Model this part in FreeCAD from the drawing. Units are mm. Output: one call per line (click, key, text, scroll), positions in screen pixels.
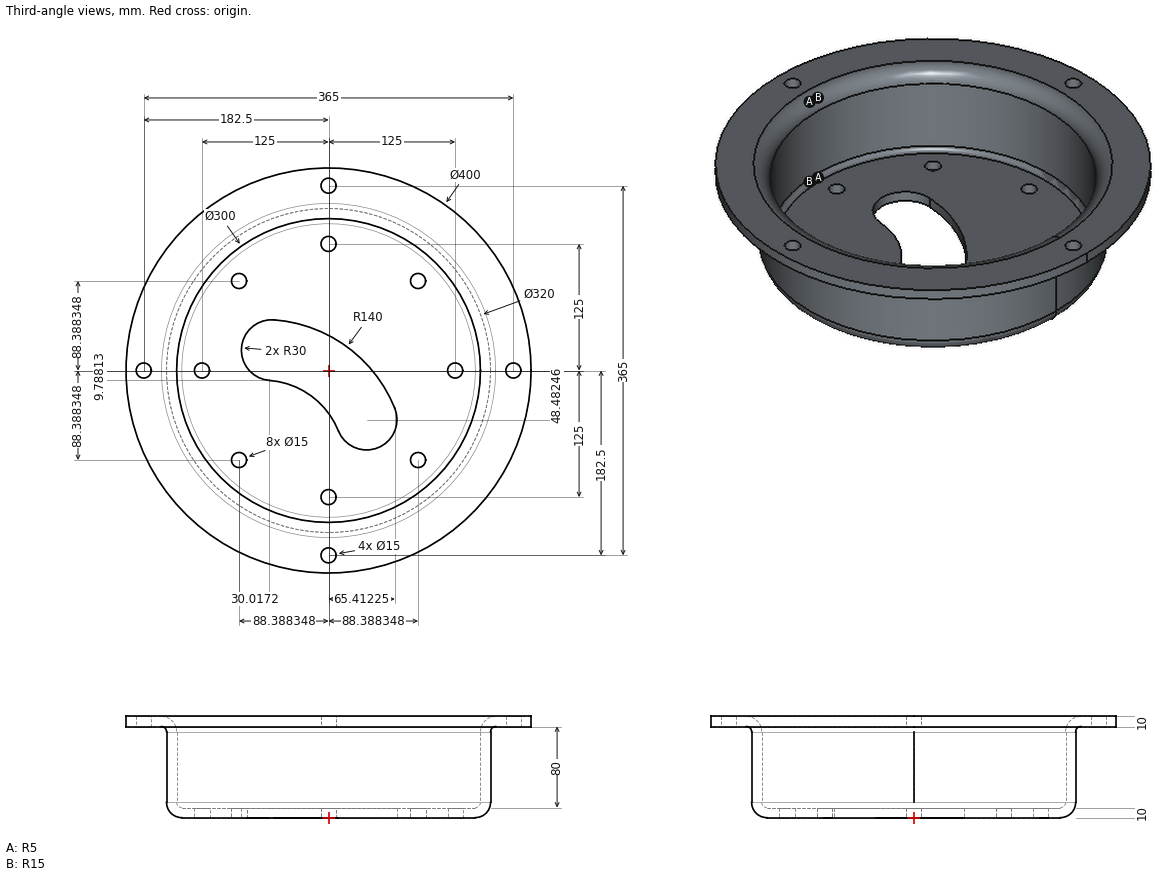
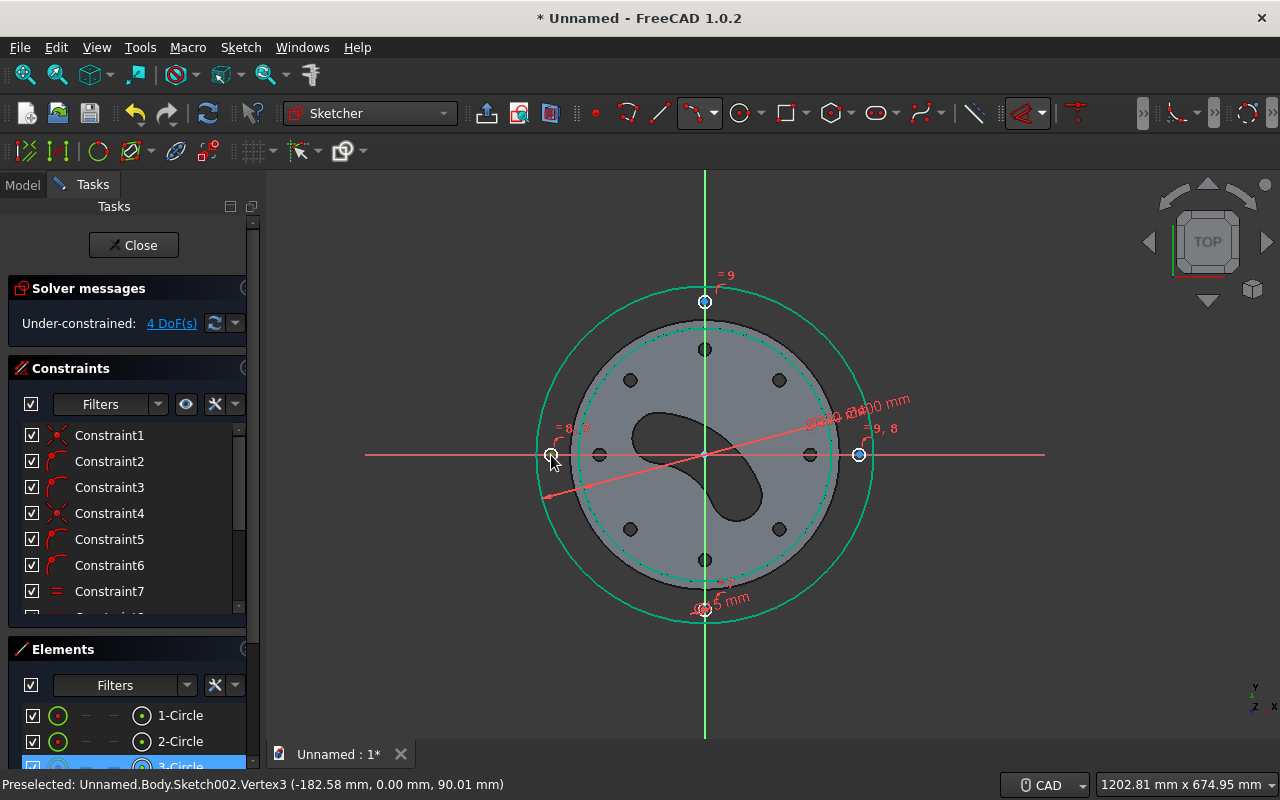
click(859, 455)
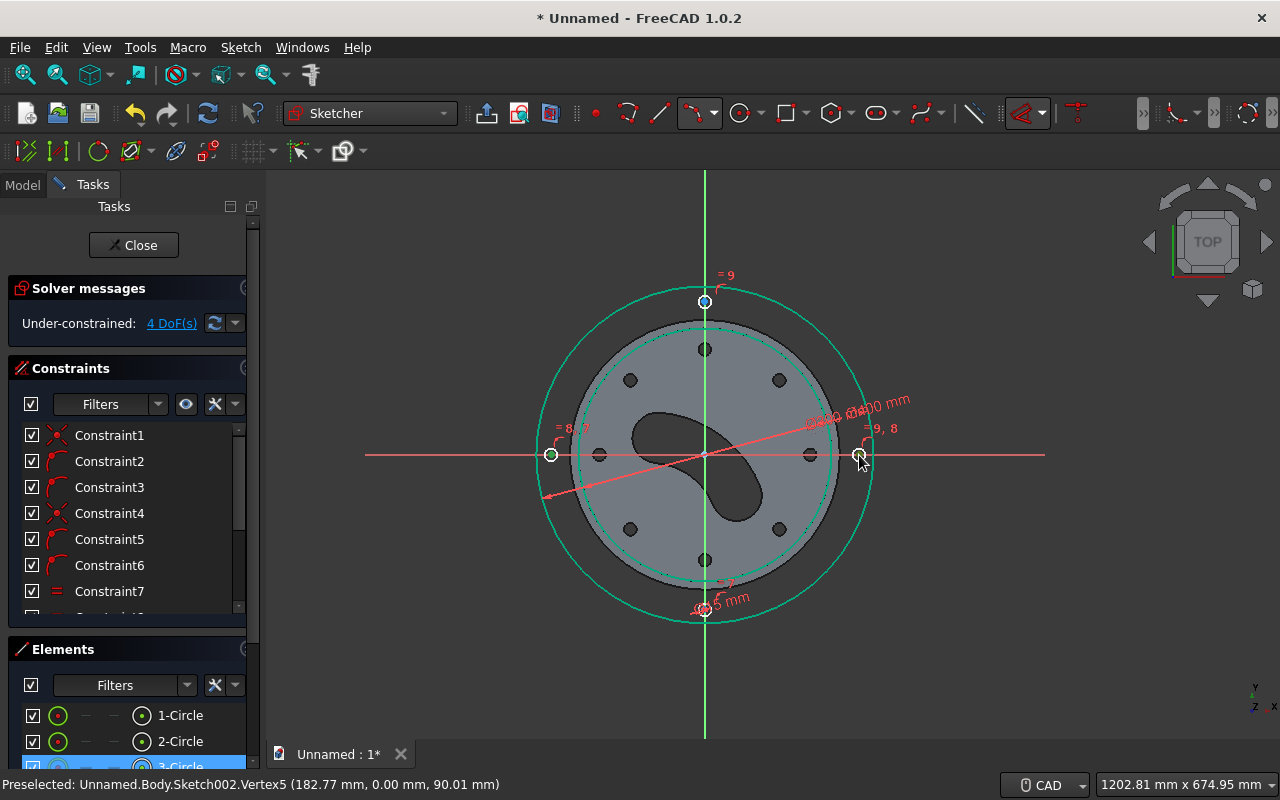
click(1044, 114)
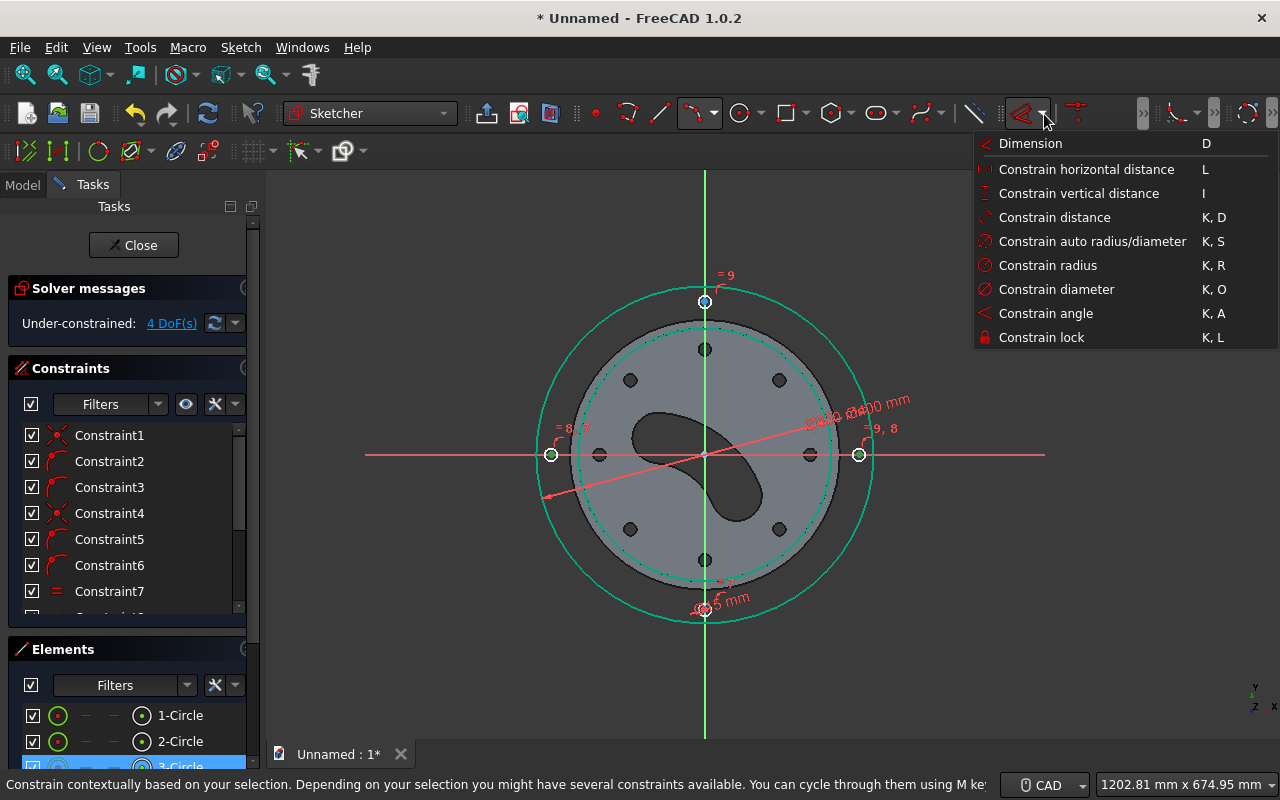
click(1126, 169)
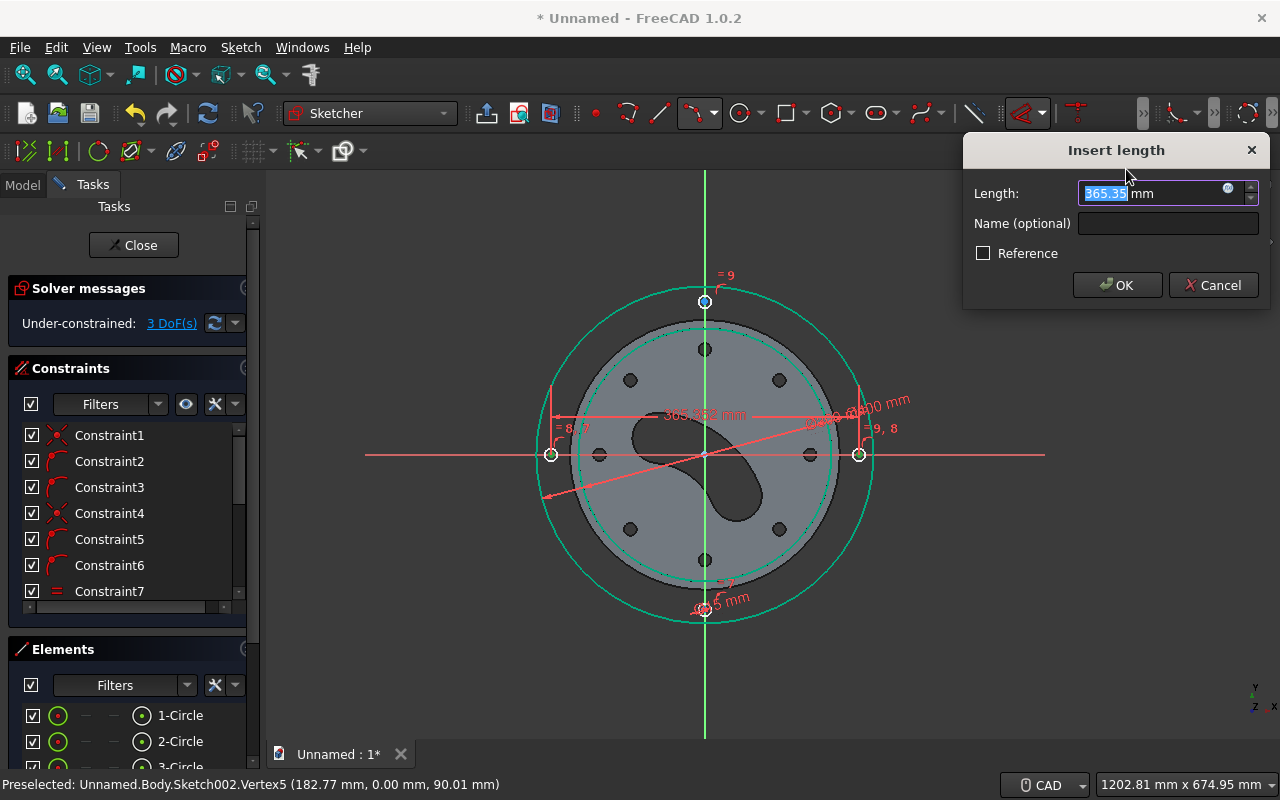
text(365)
key(Return)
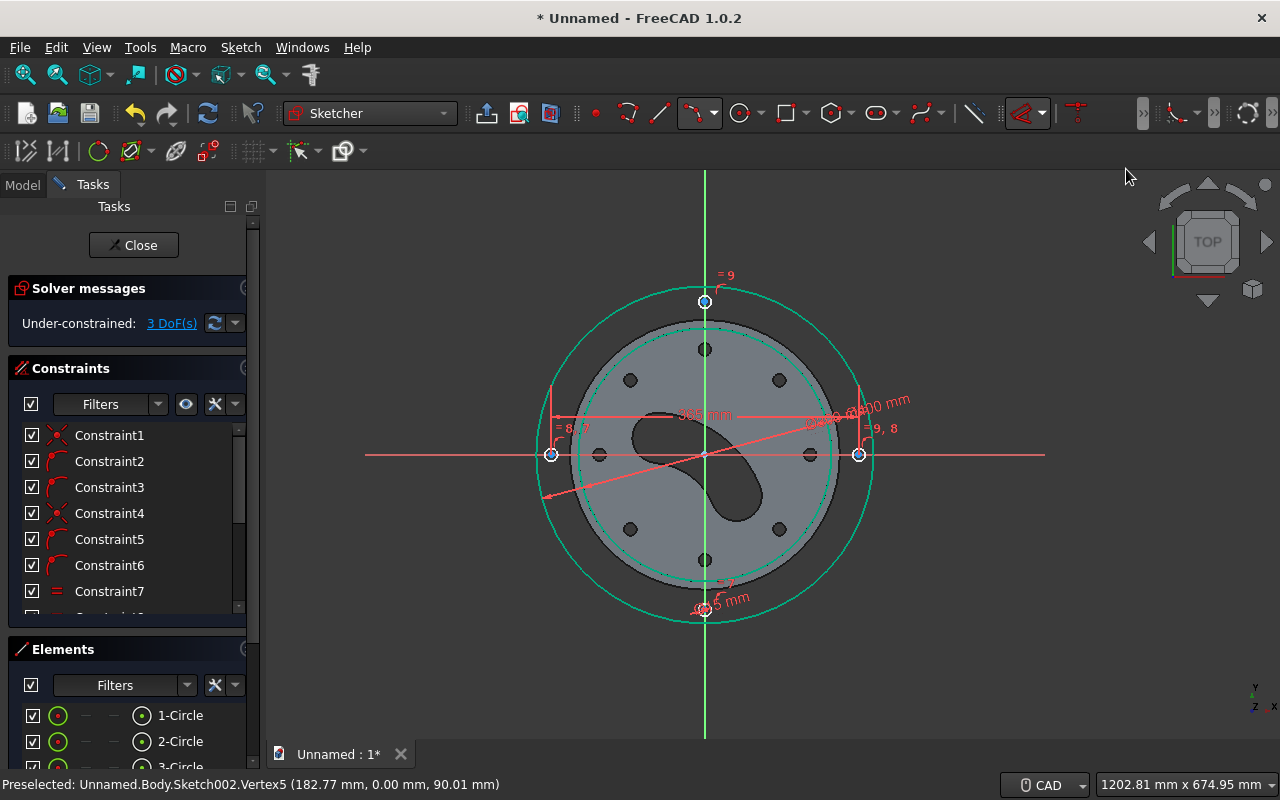
click(705, 610)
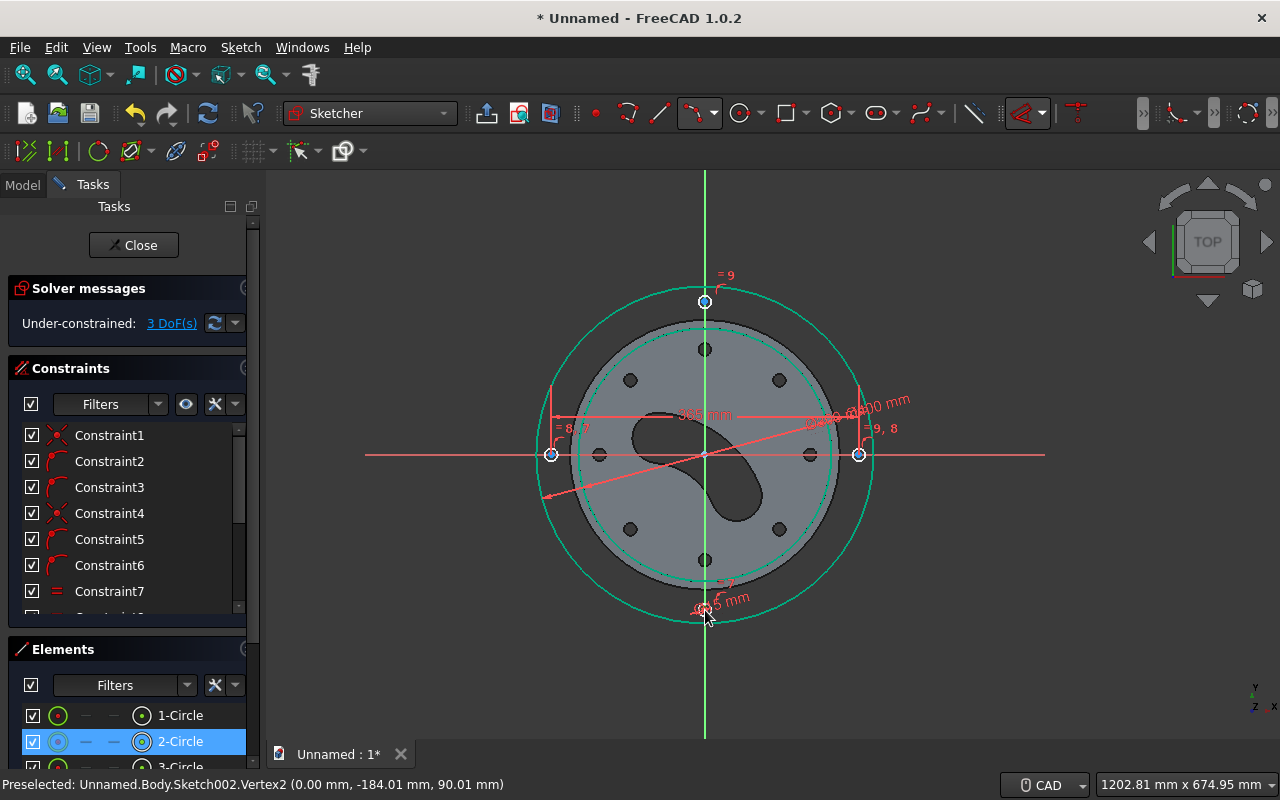
click(705, 302)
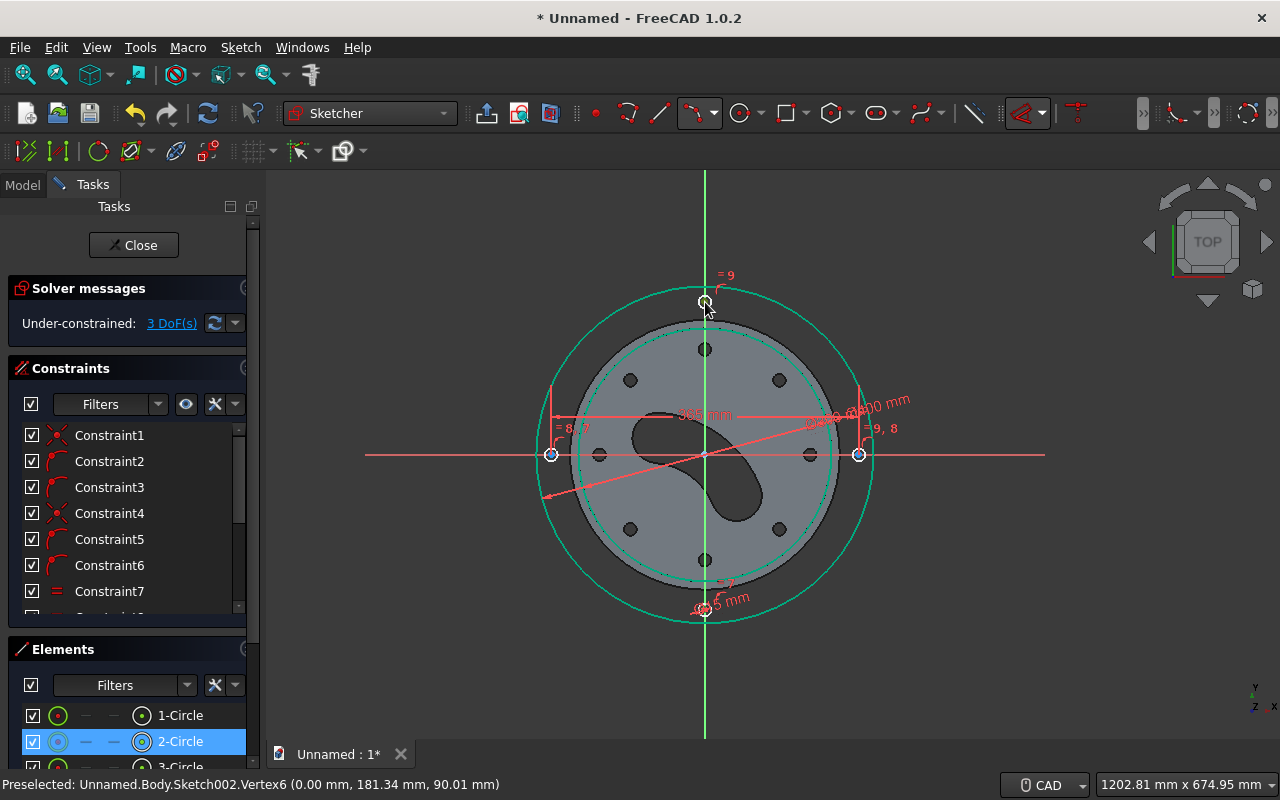
click(1044, 114)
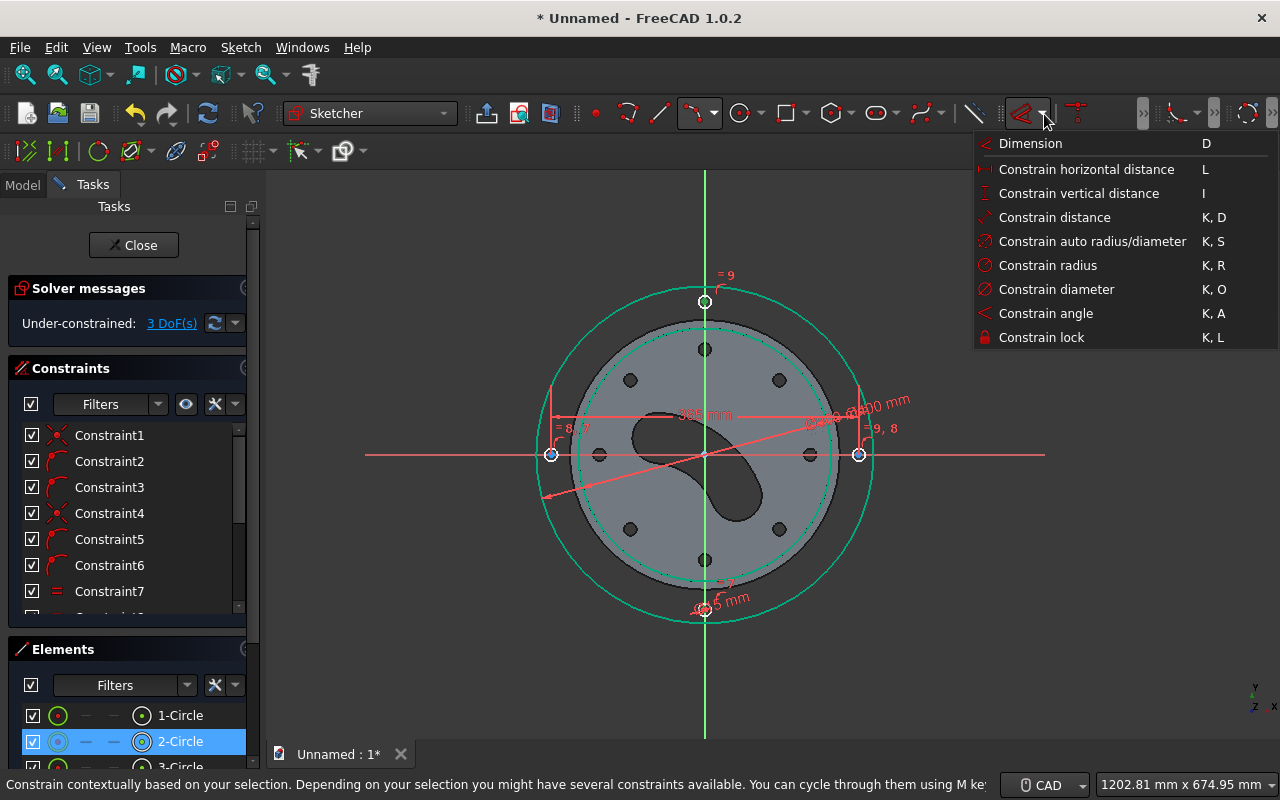
click(1126, 193)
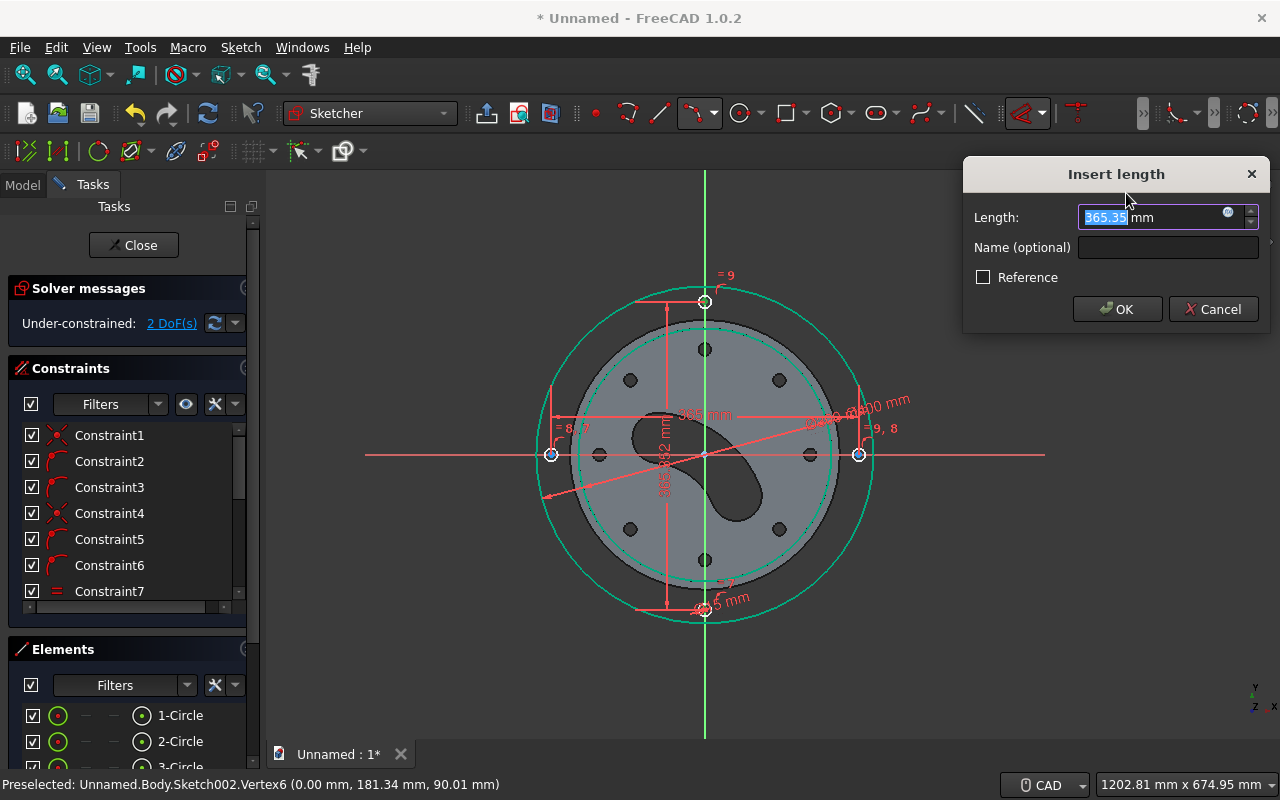
text(365)
key(Return)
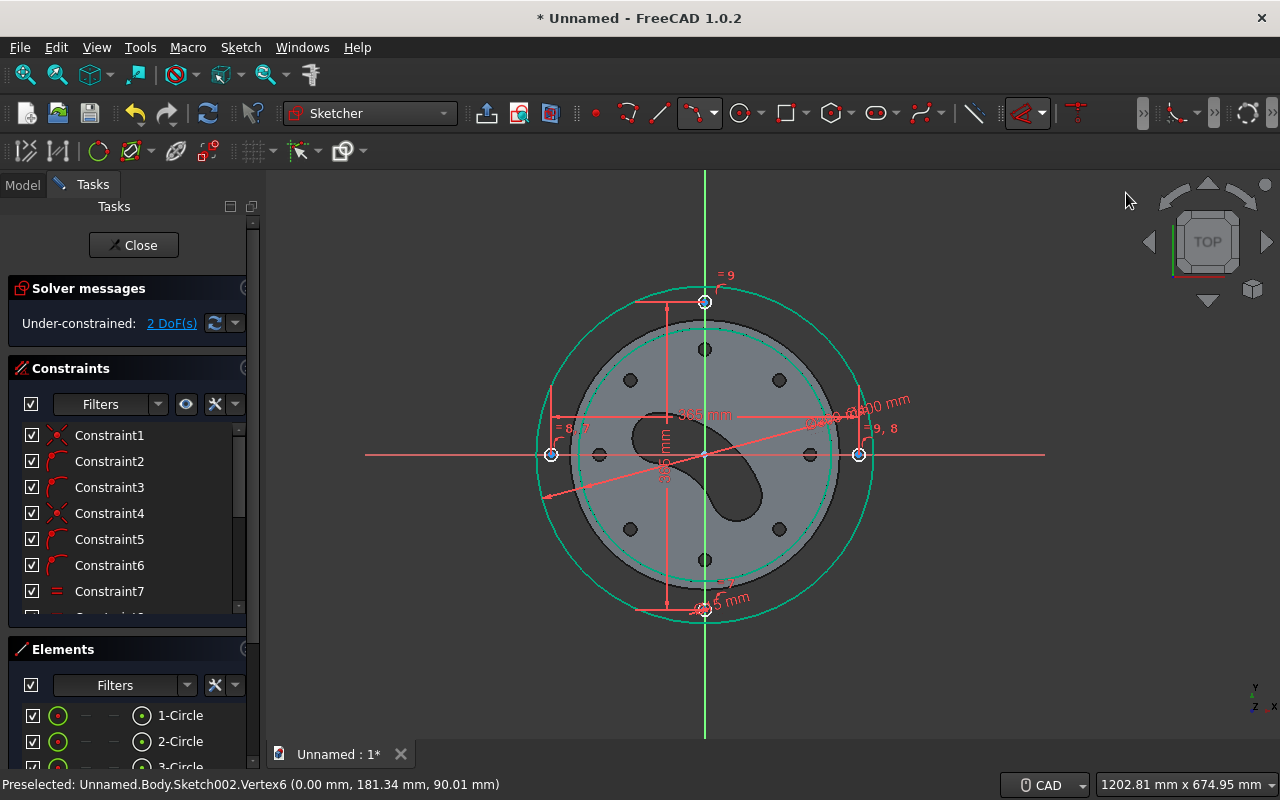
click(705, 610)